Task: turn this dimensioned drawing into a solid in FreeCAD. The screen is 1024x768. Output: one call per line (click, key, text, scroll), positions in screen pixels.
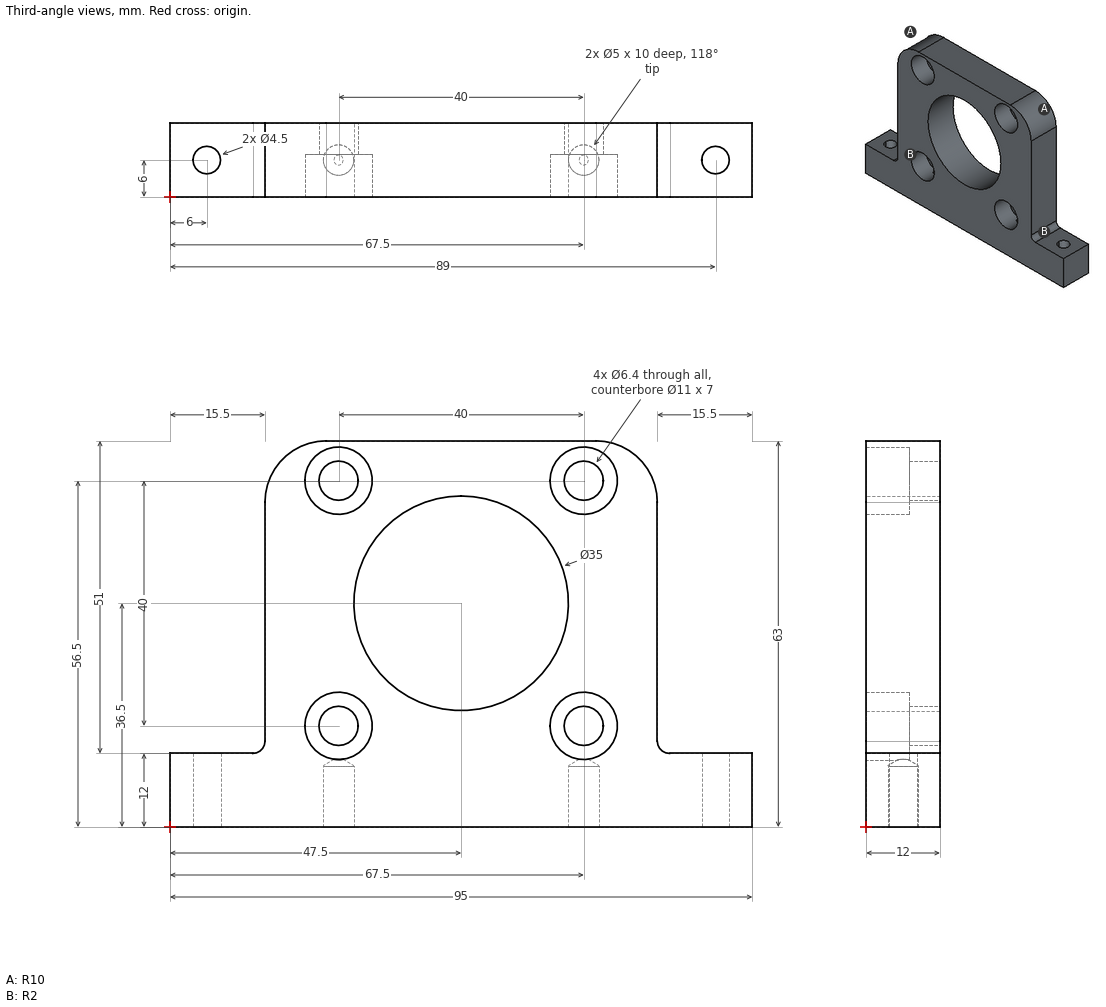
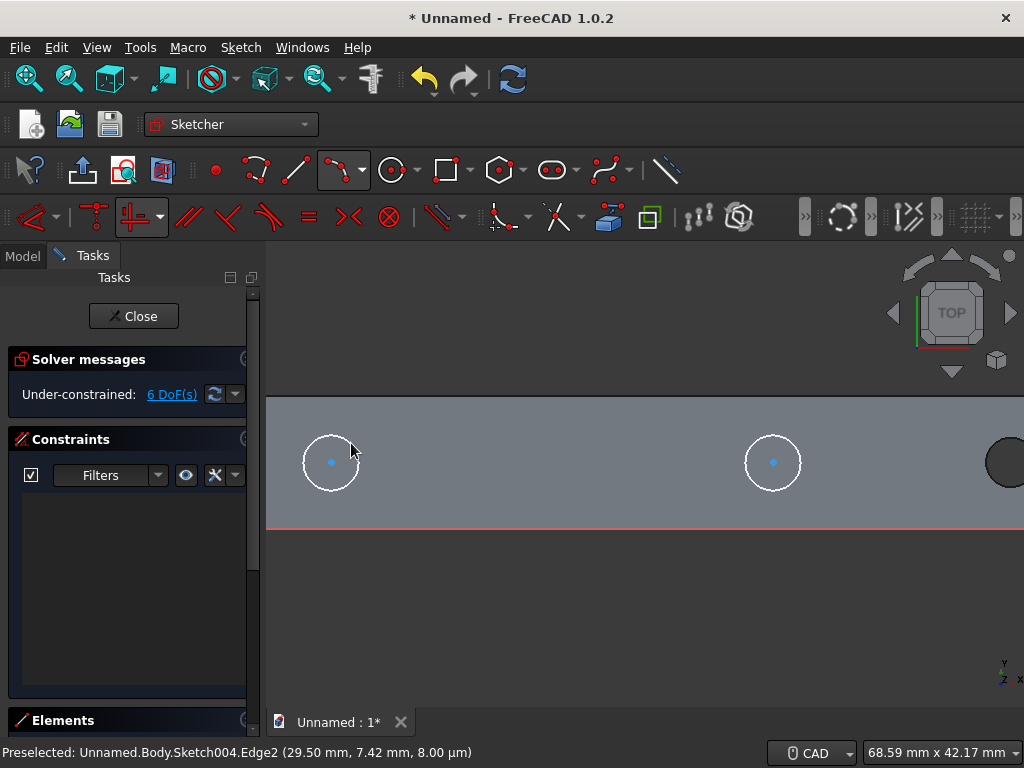
click(792, 443)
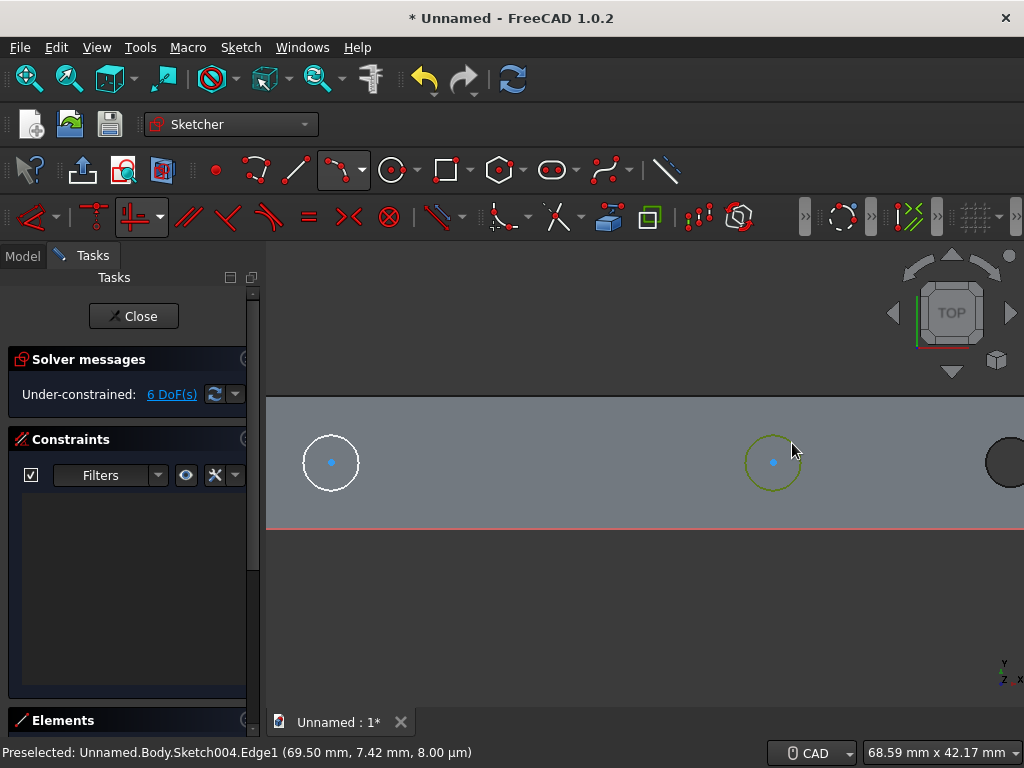
click(350, 443)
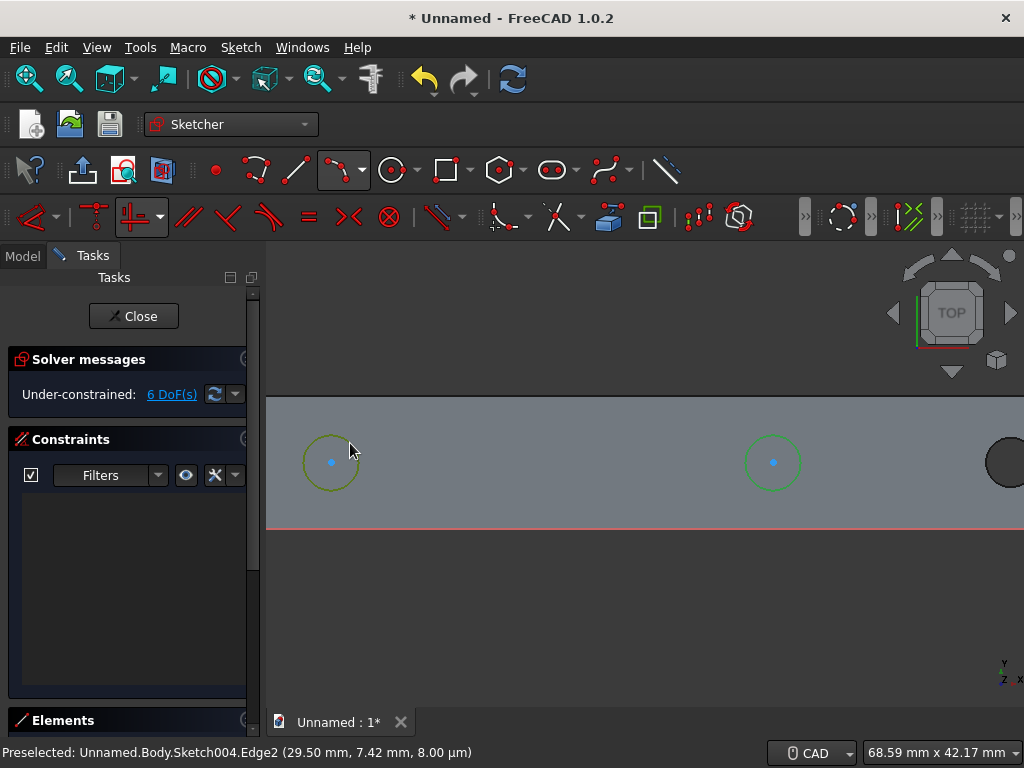
click(310, 218)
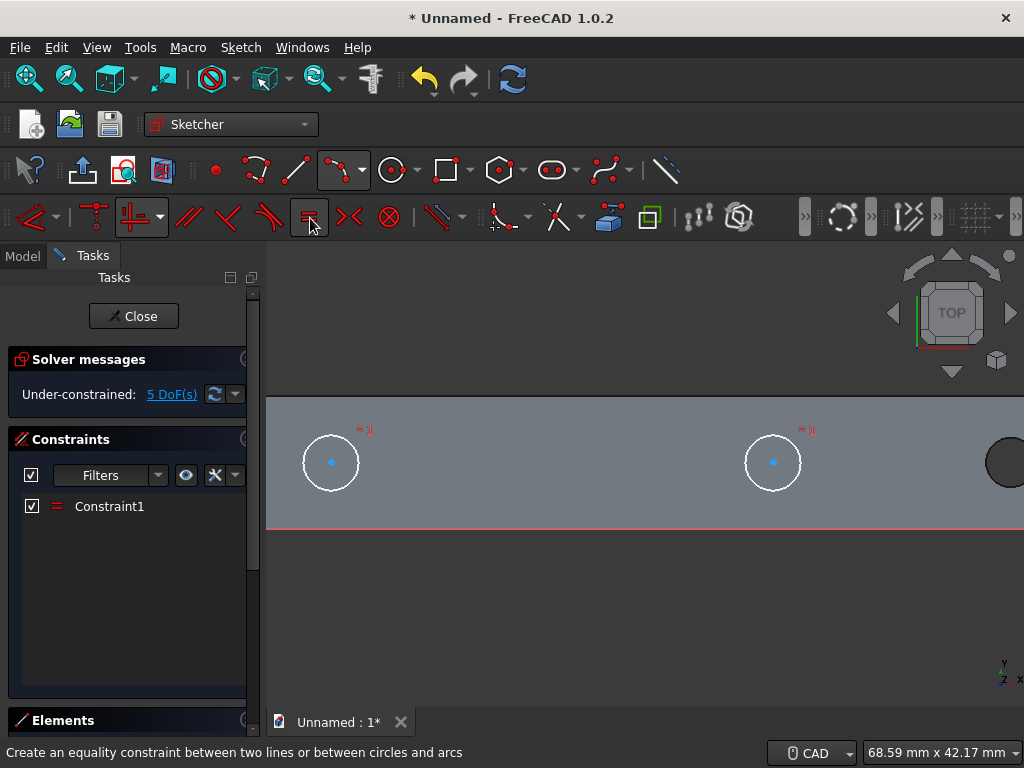
click(773, 463)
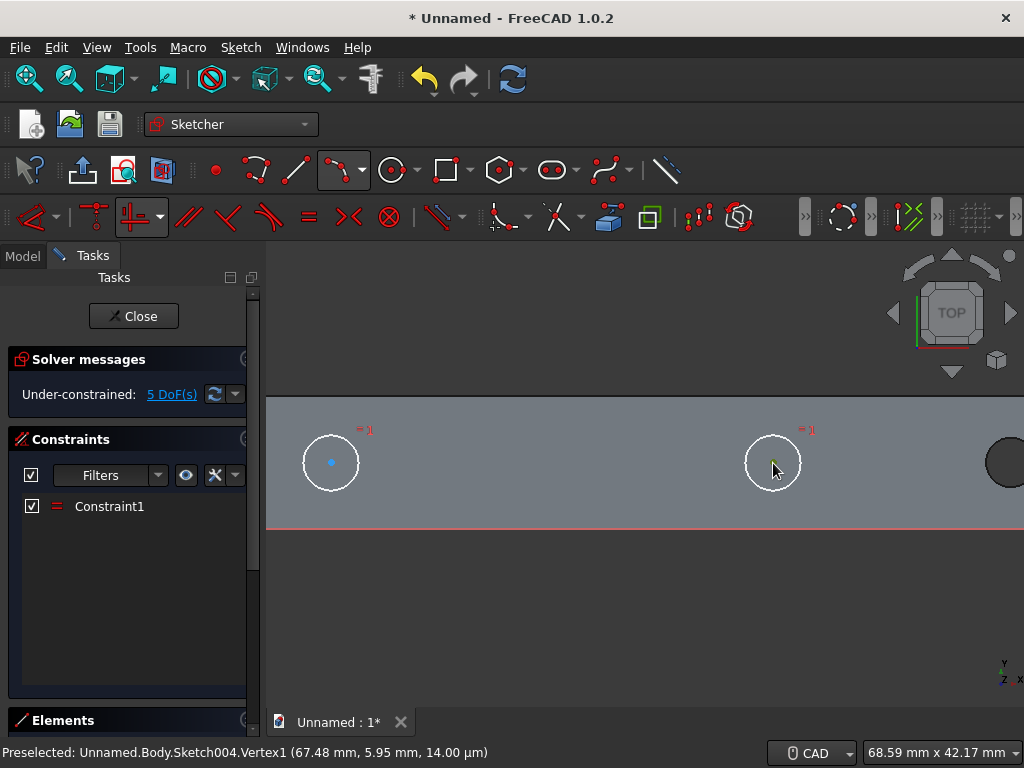
click(331, 463)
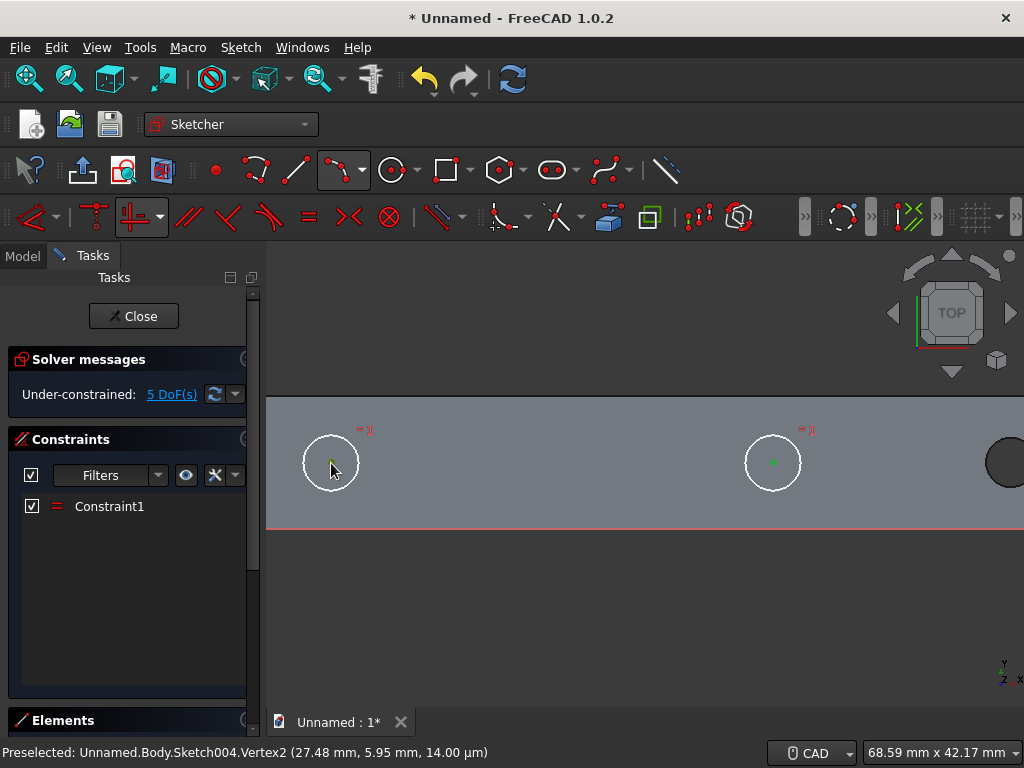
click(162, 218)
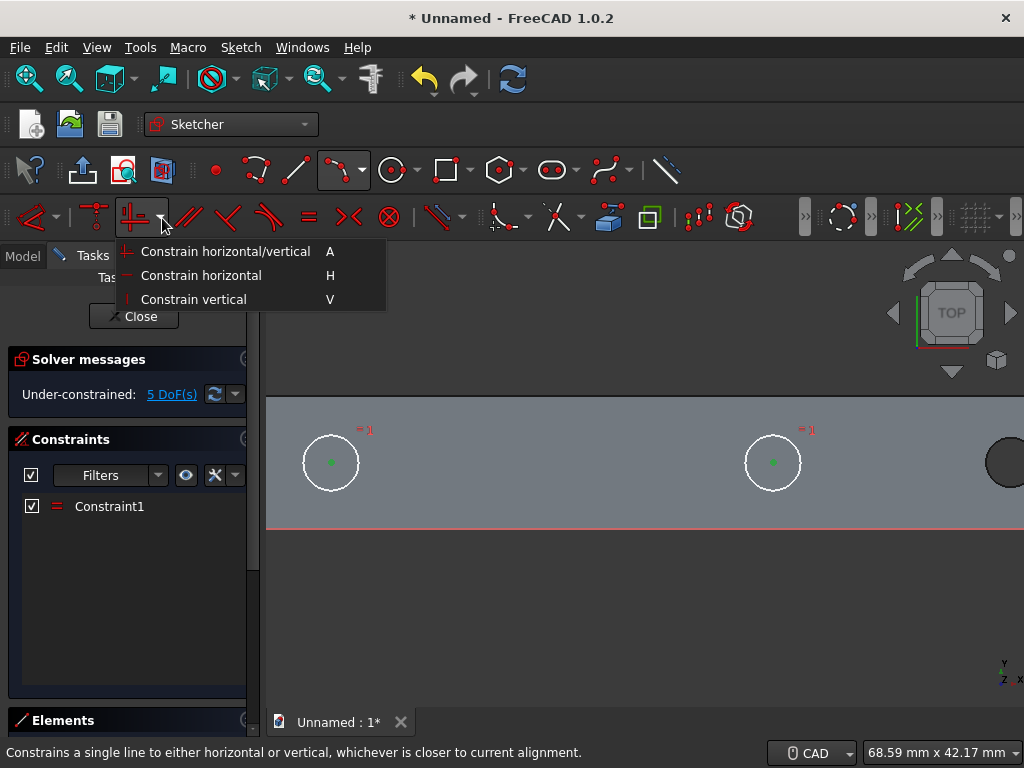
click(251, 275)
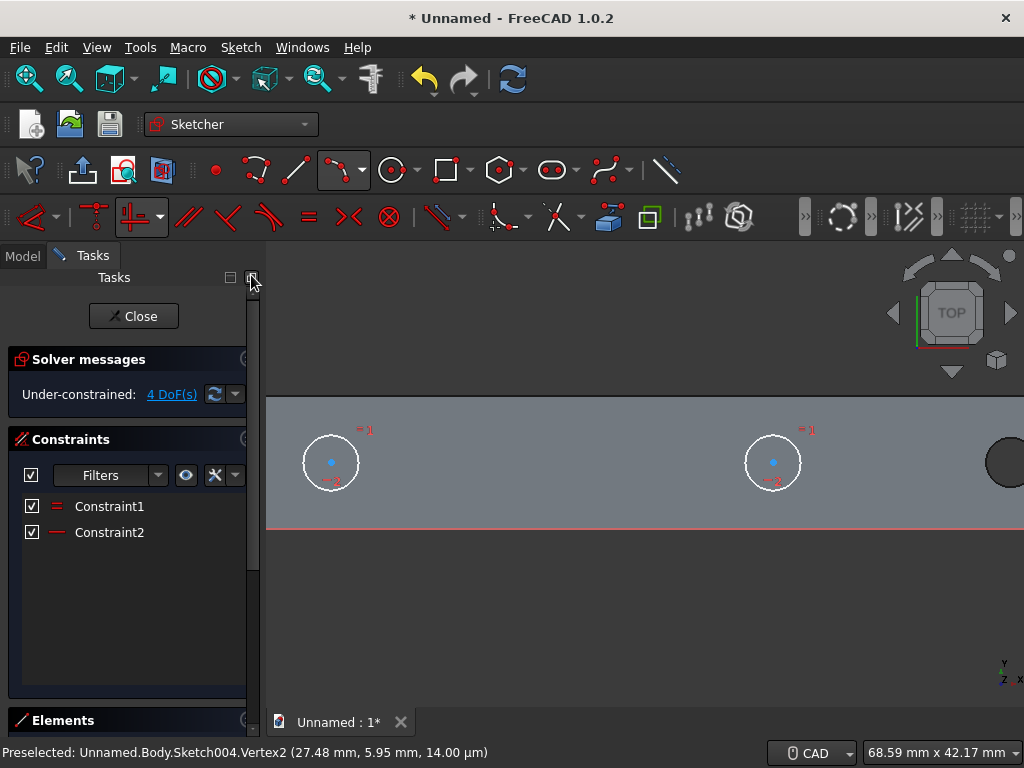
click(32, 218)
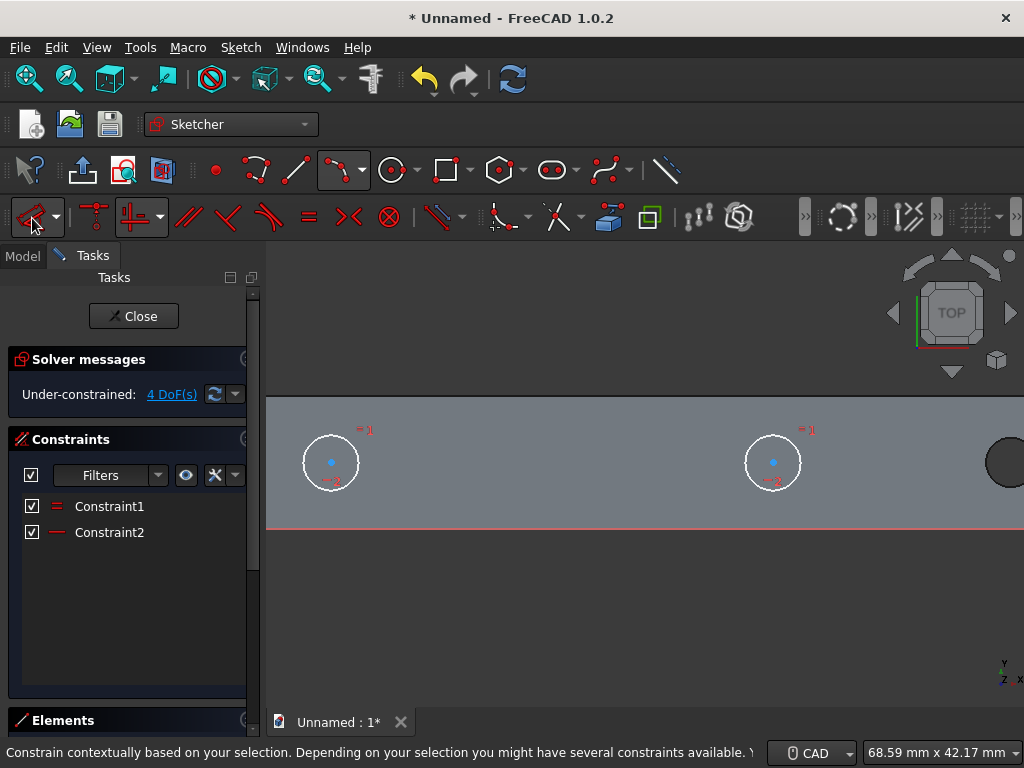
click(792, 443)
click(814, 420)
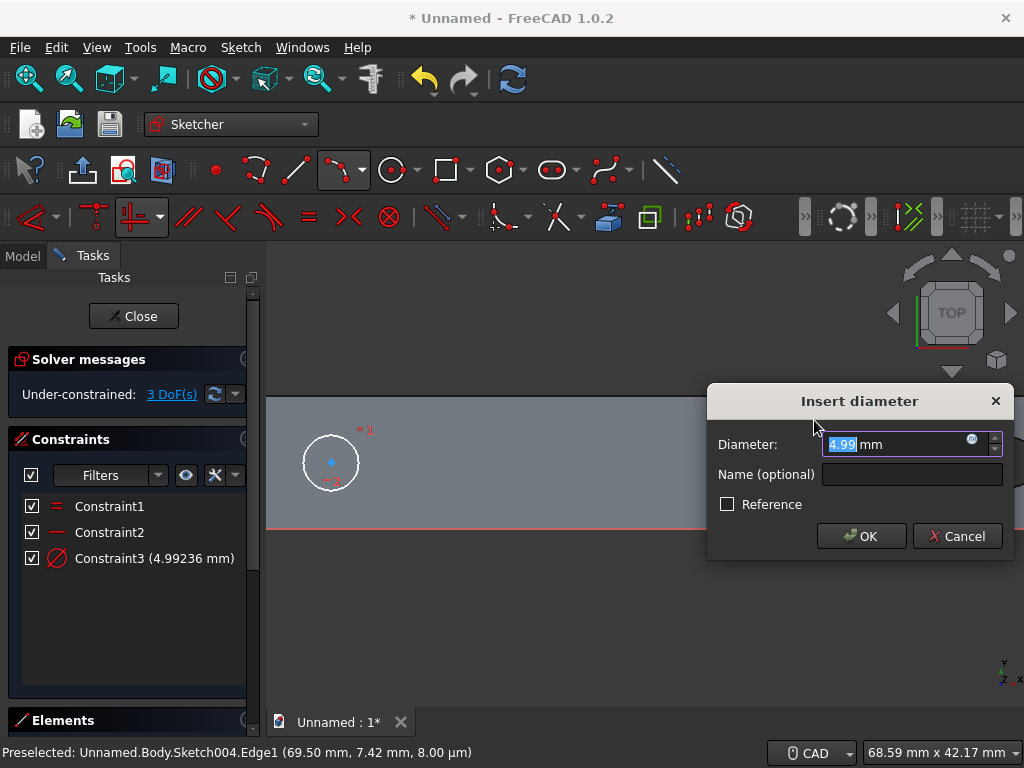
text(5)
key(Return)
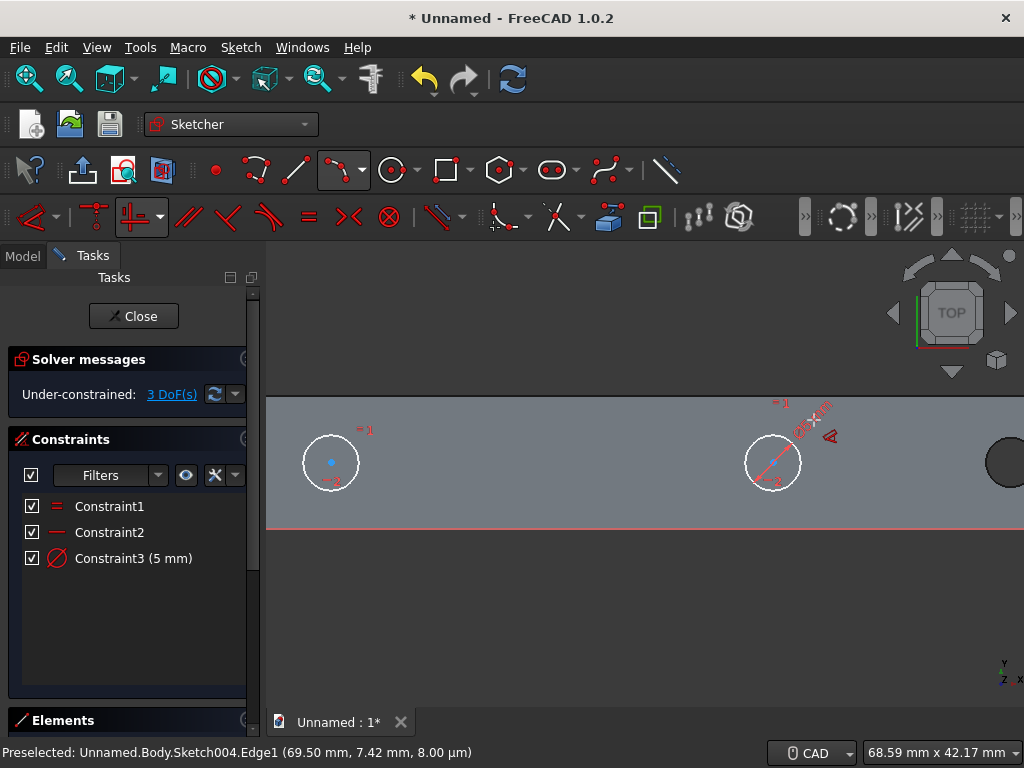
click(773, 463)
click(807, 496)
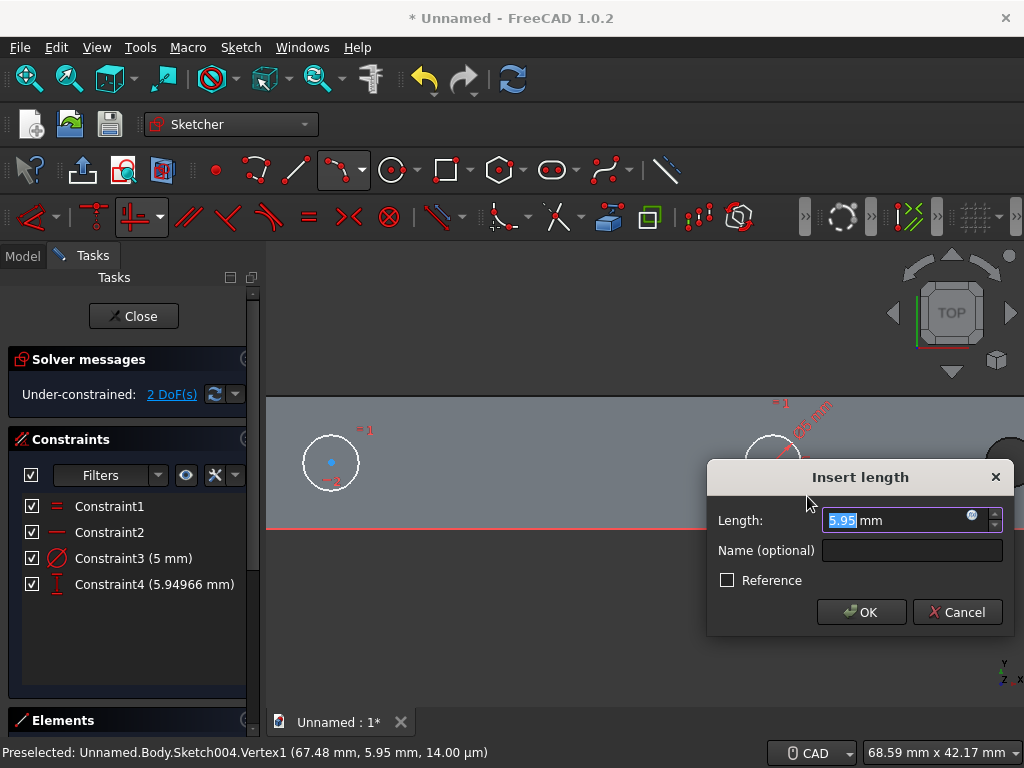
text(6)
key(Return)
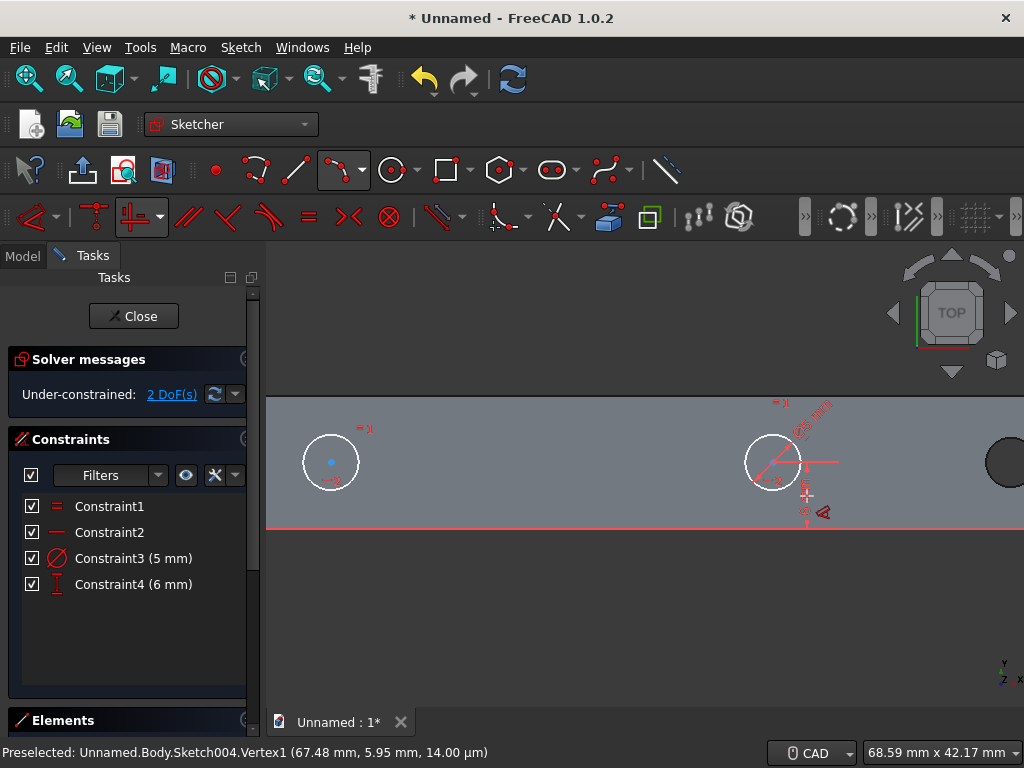
click(773, 462)